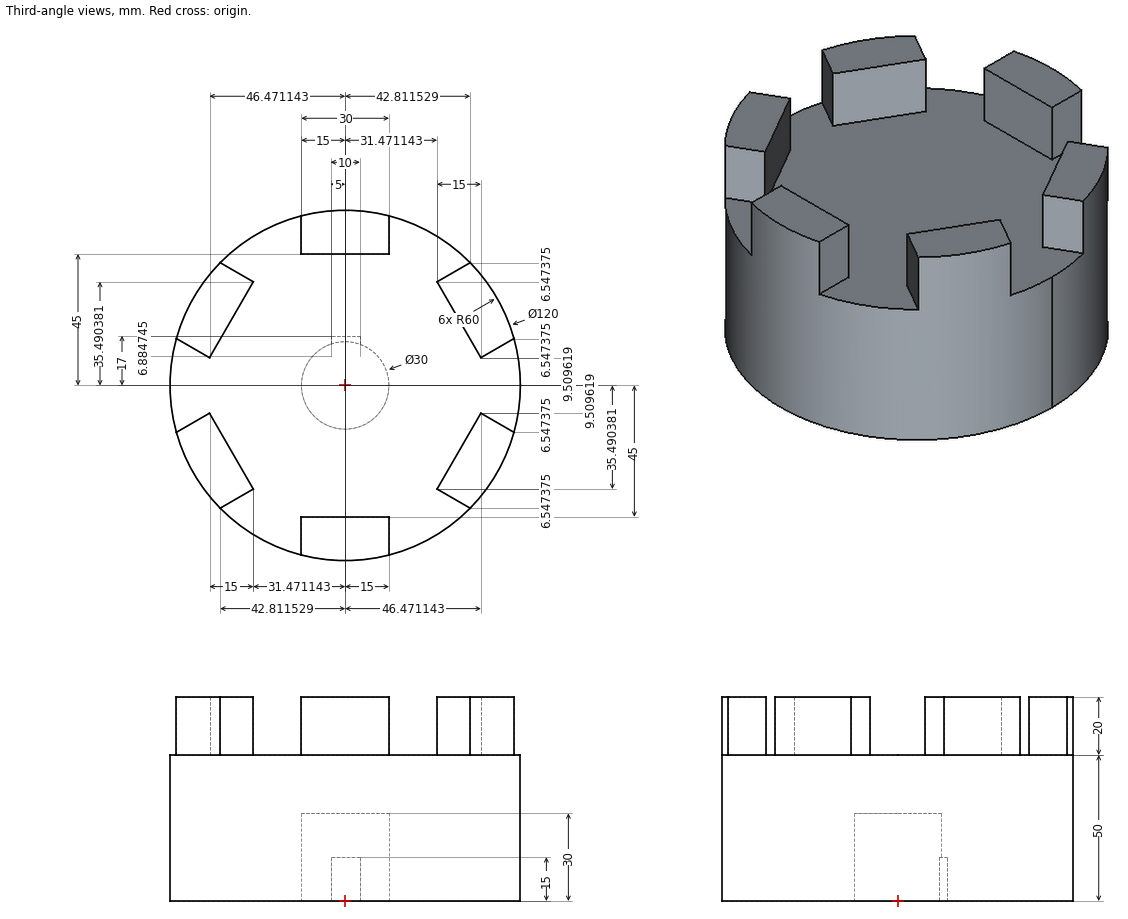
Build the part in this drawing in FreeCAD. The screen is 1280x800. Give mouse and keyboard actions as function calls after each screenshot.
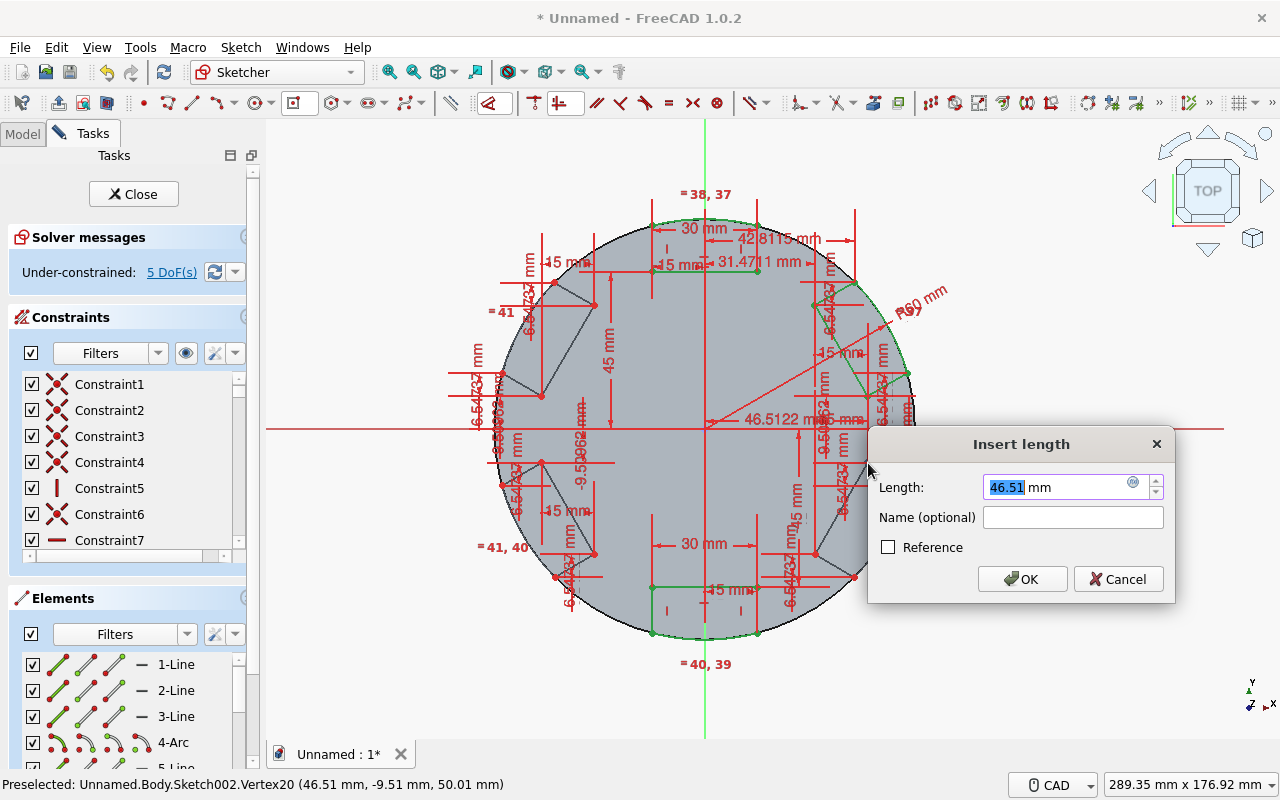
text(46.471143)
key(Return)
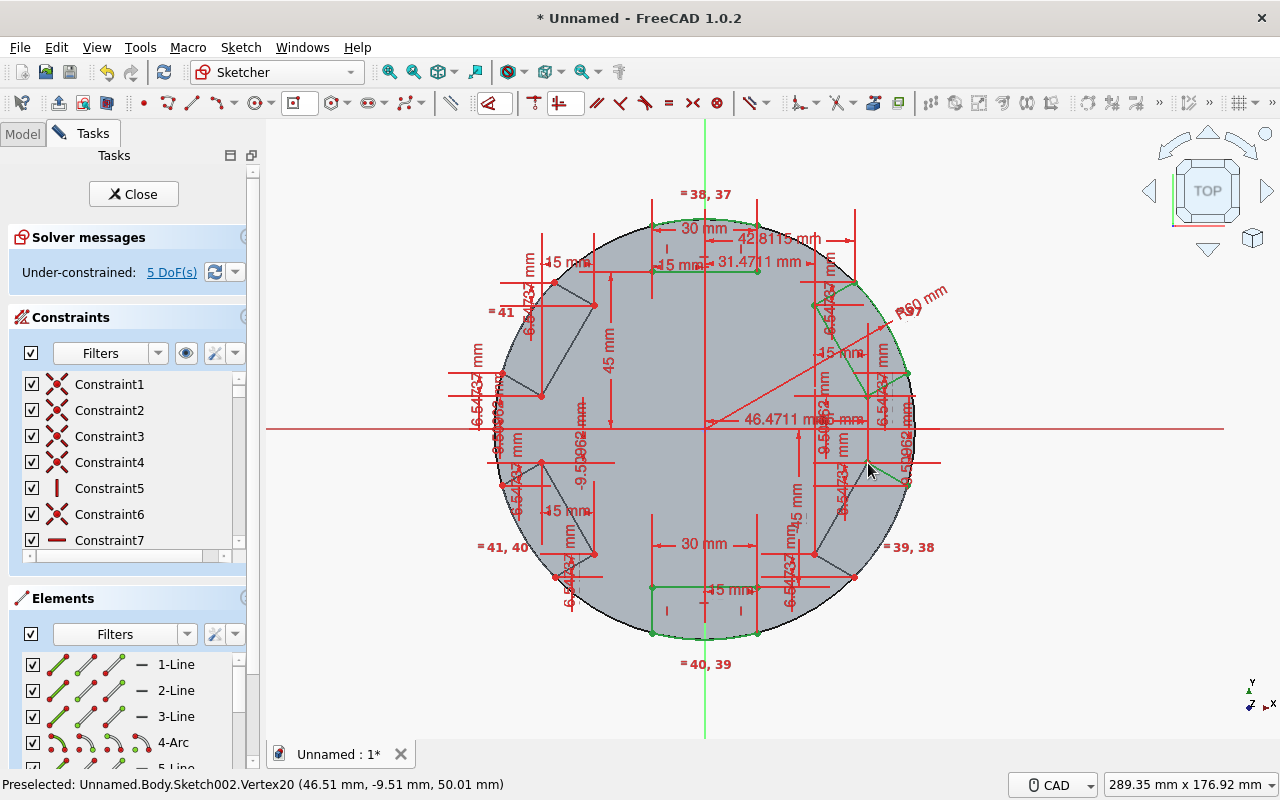
click(815, 554)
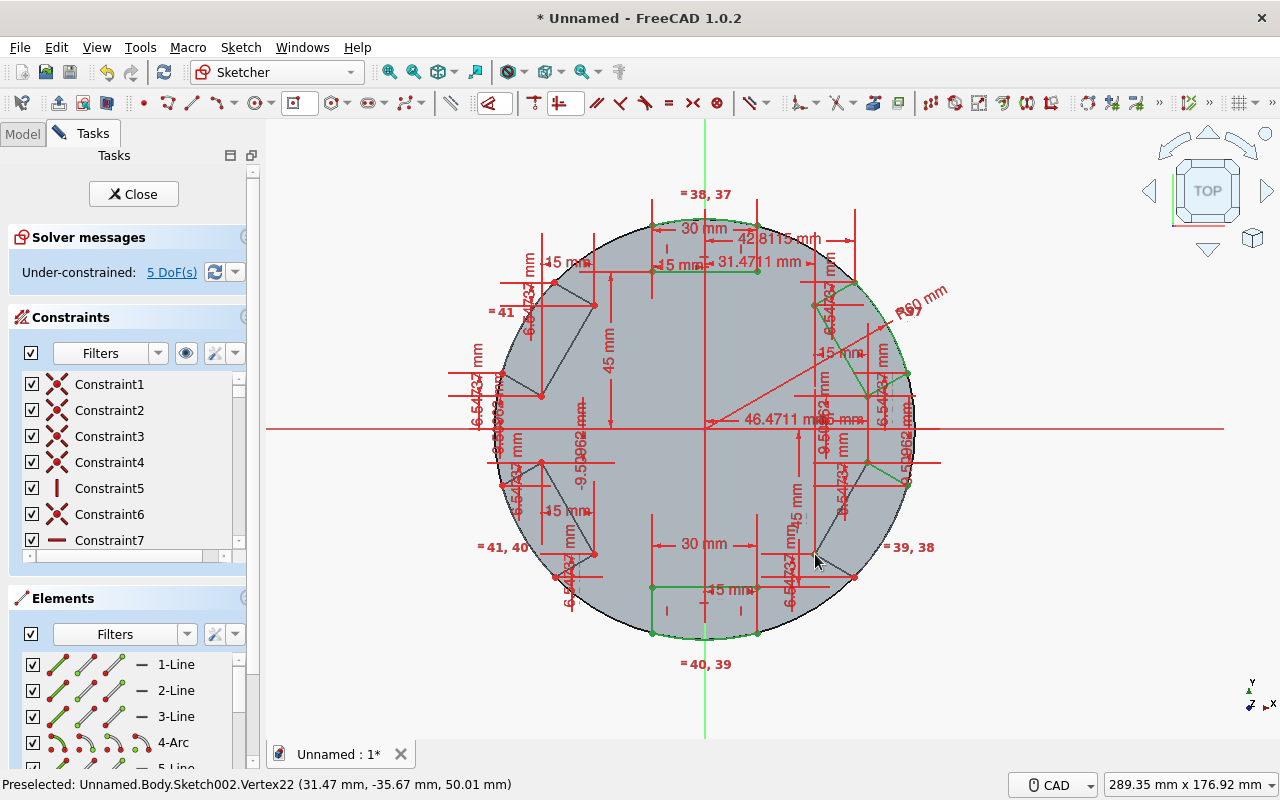
key(i)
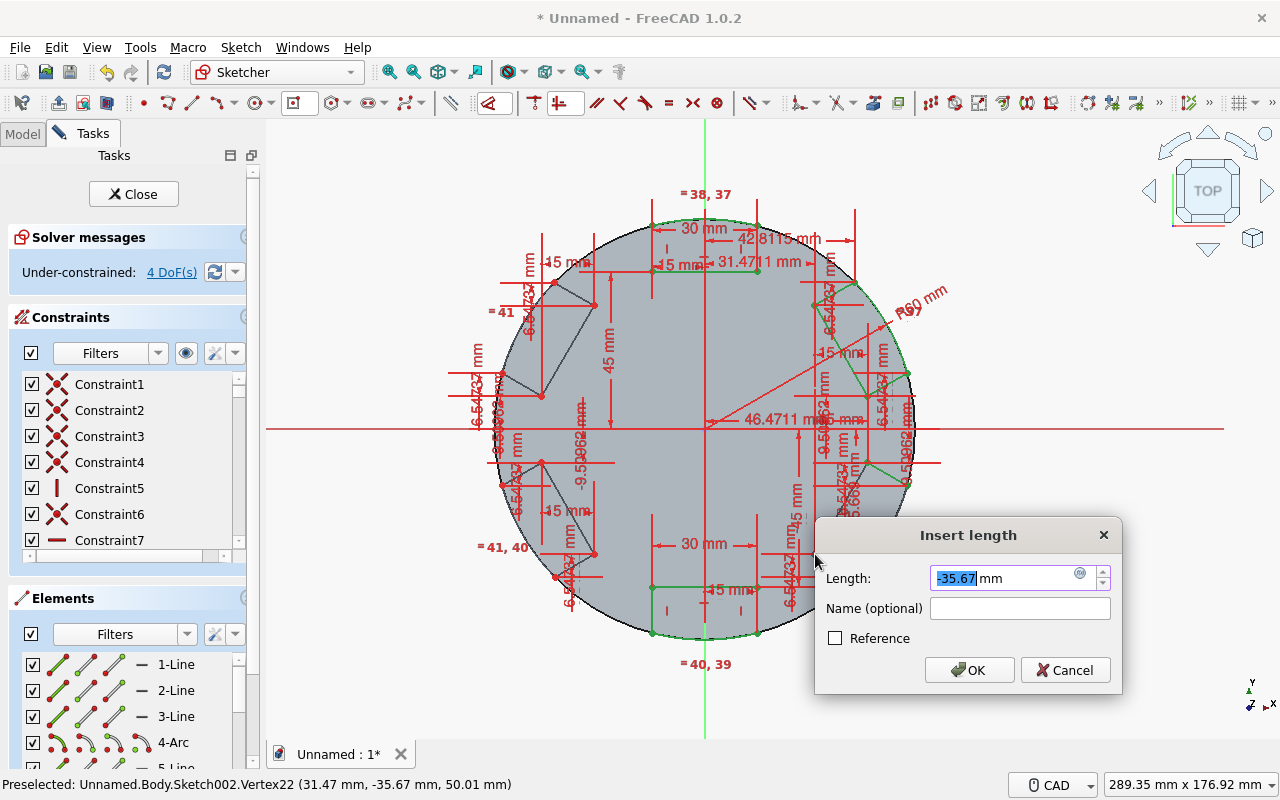
text(-35.490381)
key(Return)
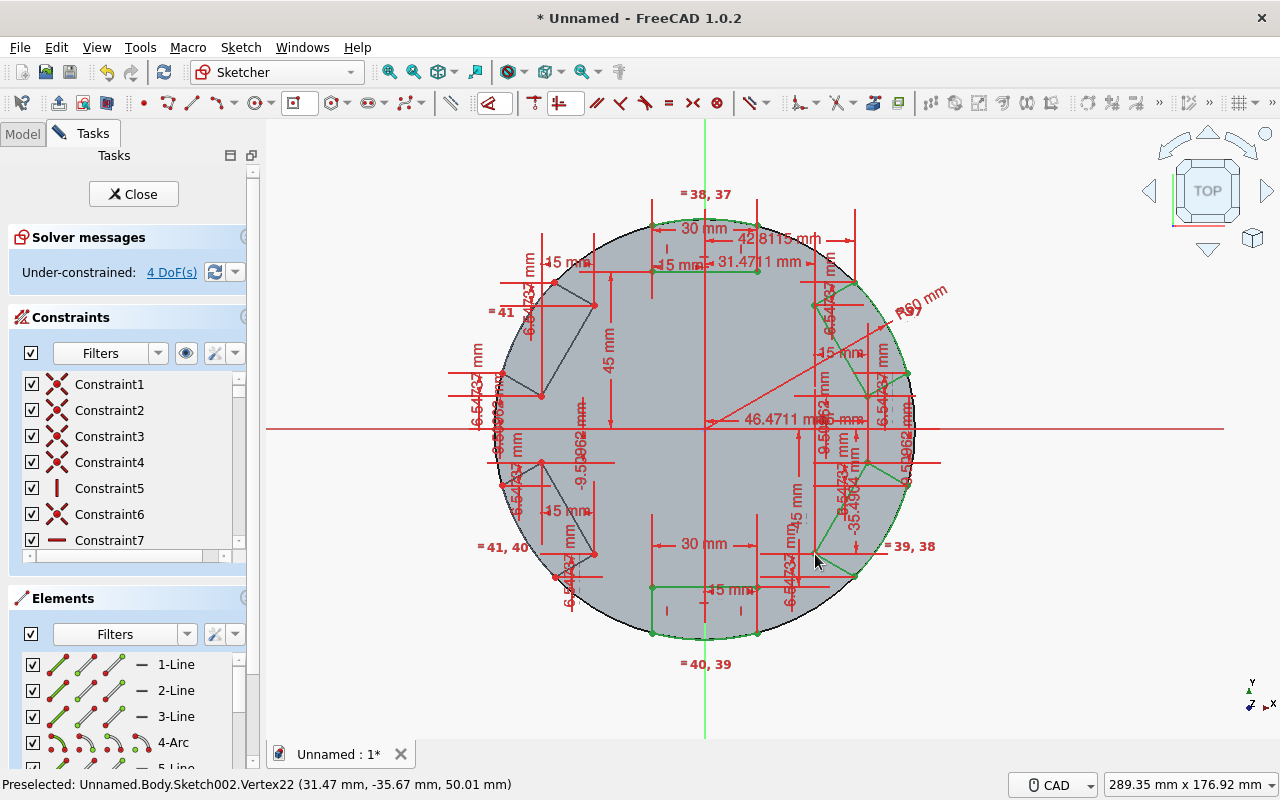
click(555, 577)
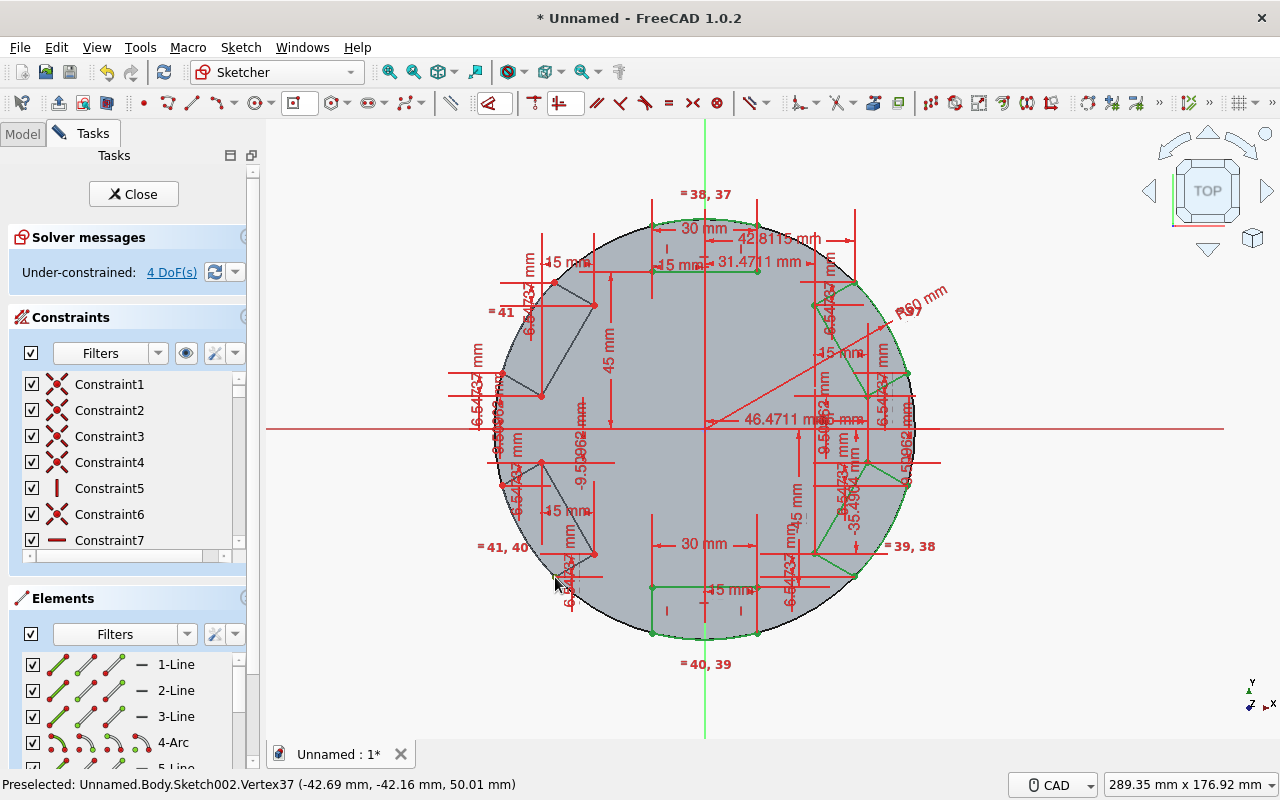
key(l)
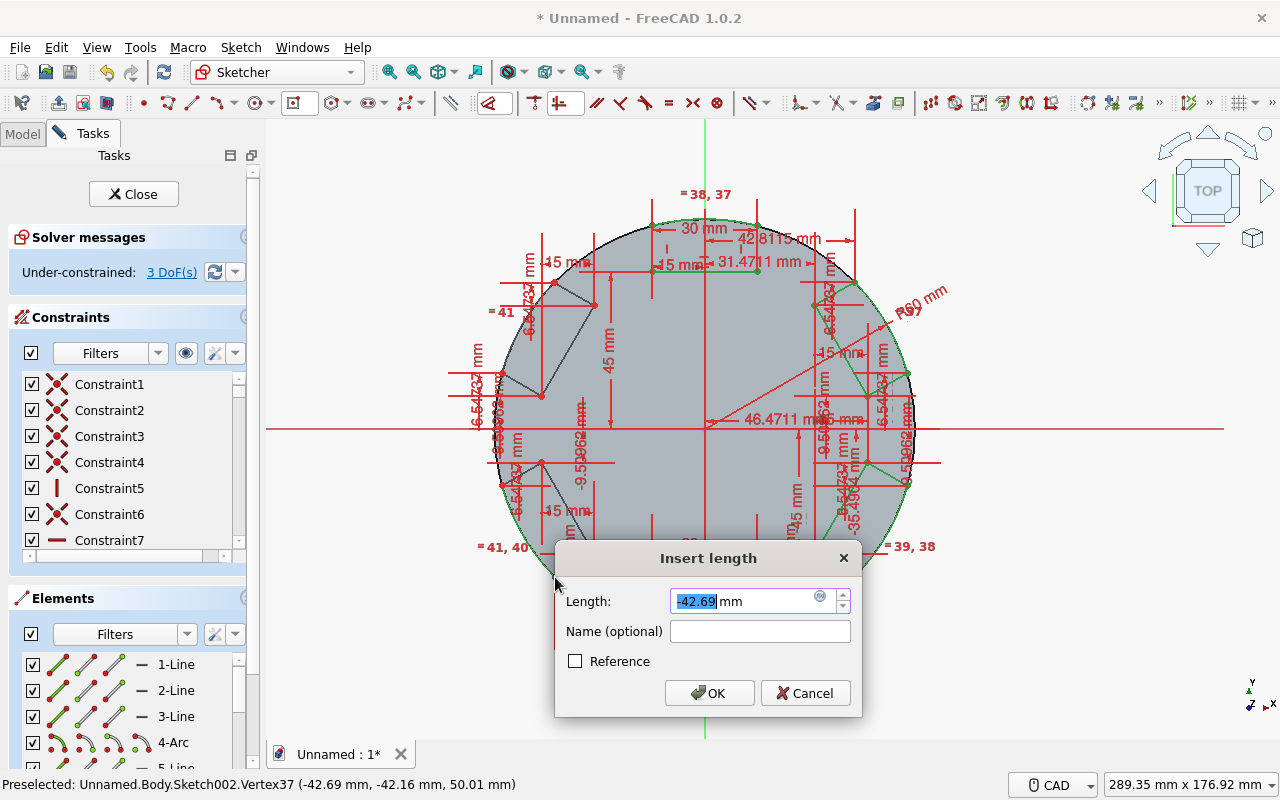
text(-42.811529)
key(Return)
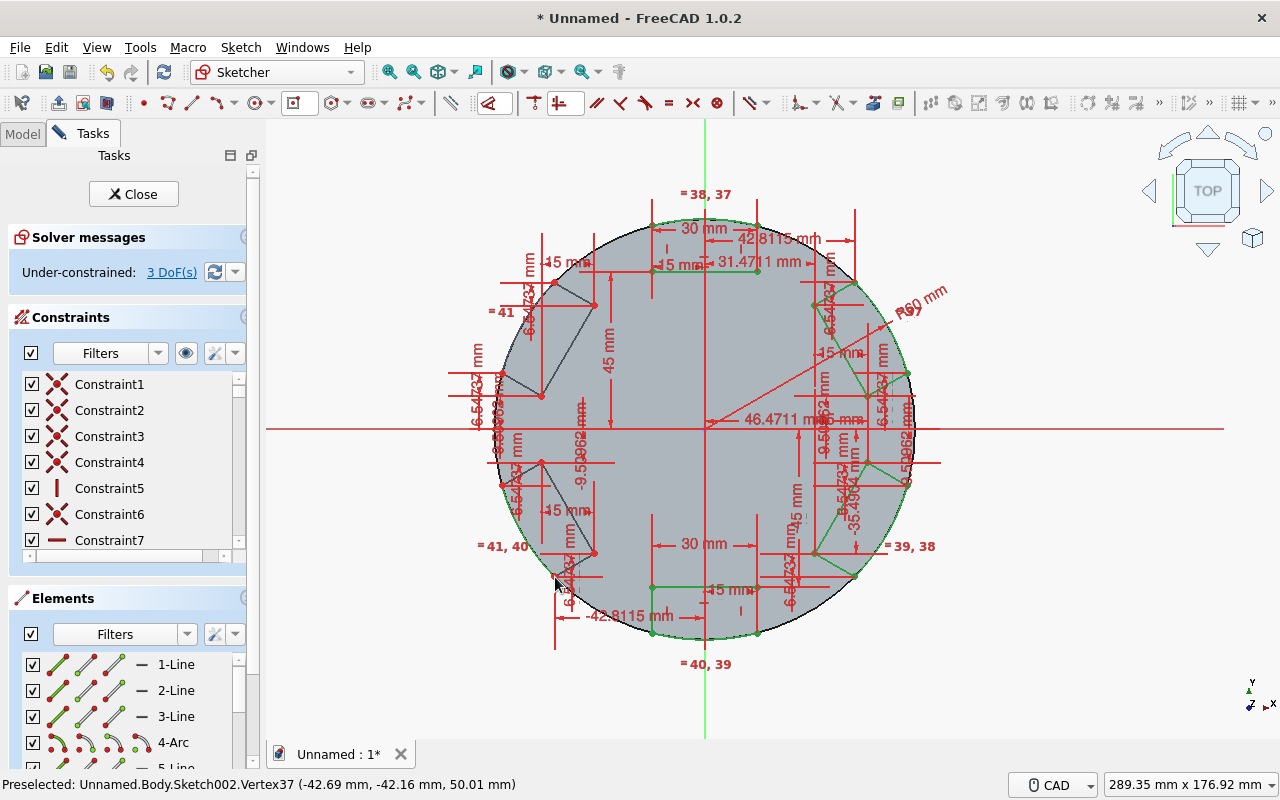
click(594, 554)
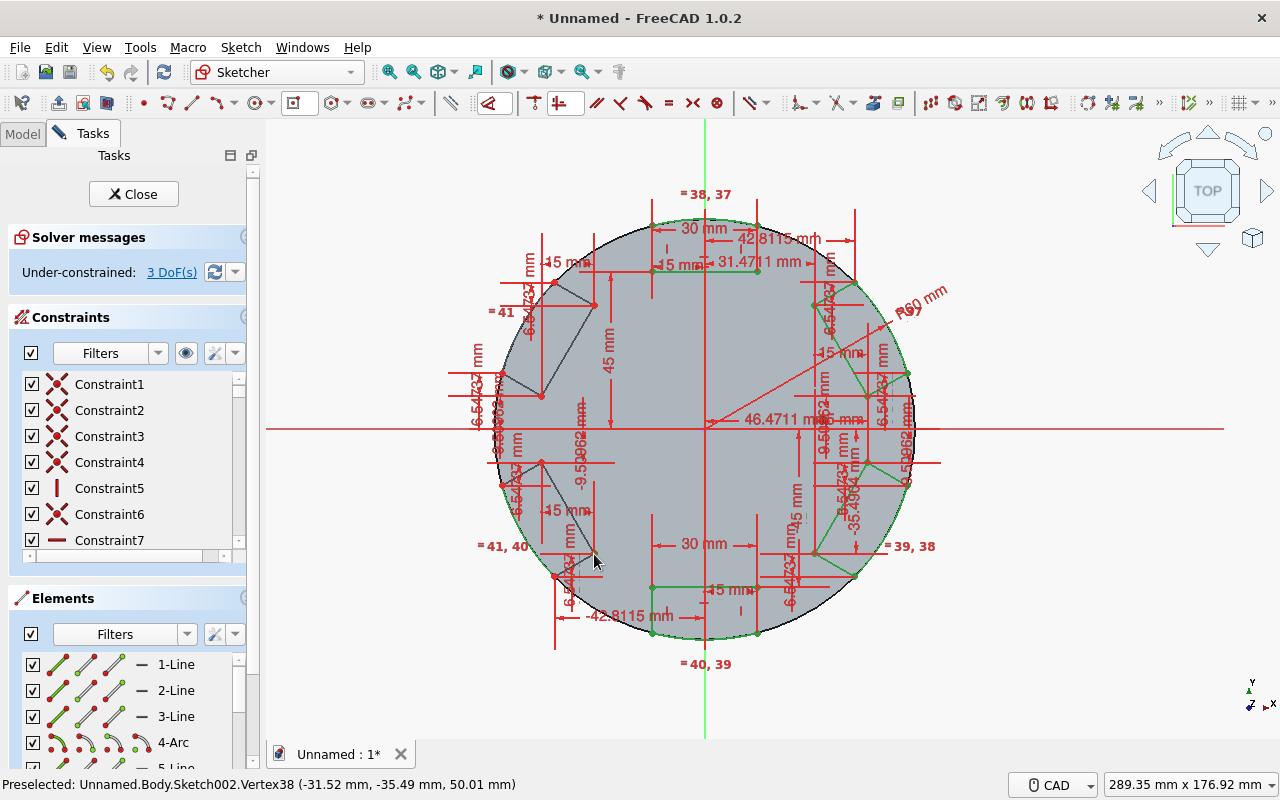
click(506, 104)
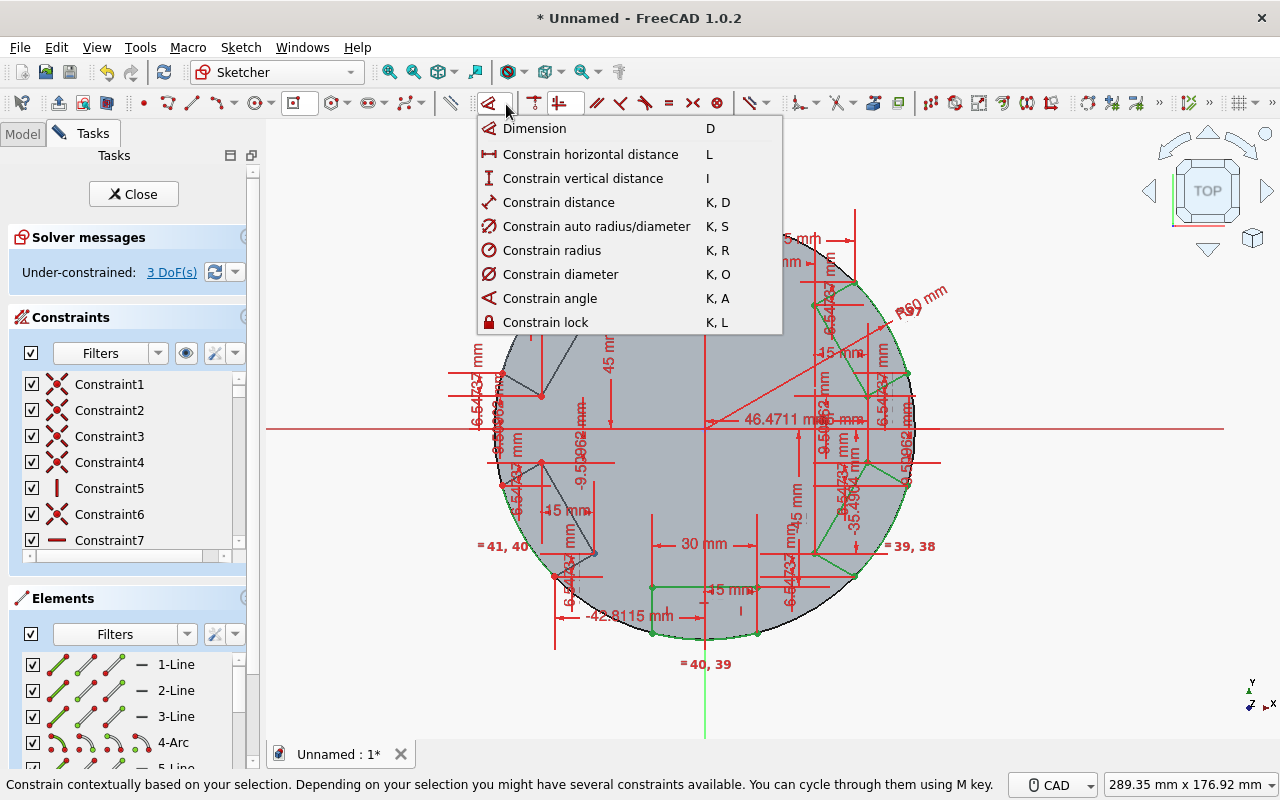
click(630, 154)